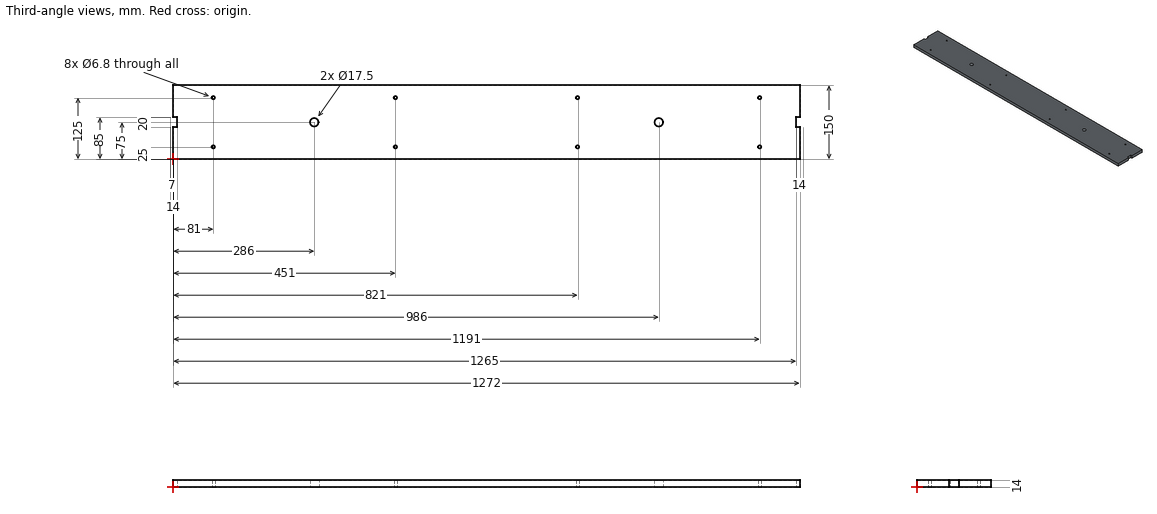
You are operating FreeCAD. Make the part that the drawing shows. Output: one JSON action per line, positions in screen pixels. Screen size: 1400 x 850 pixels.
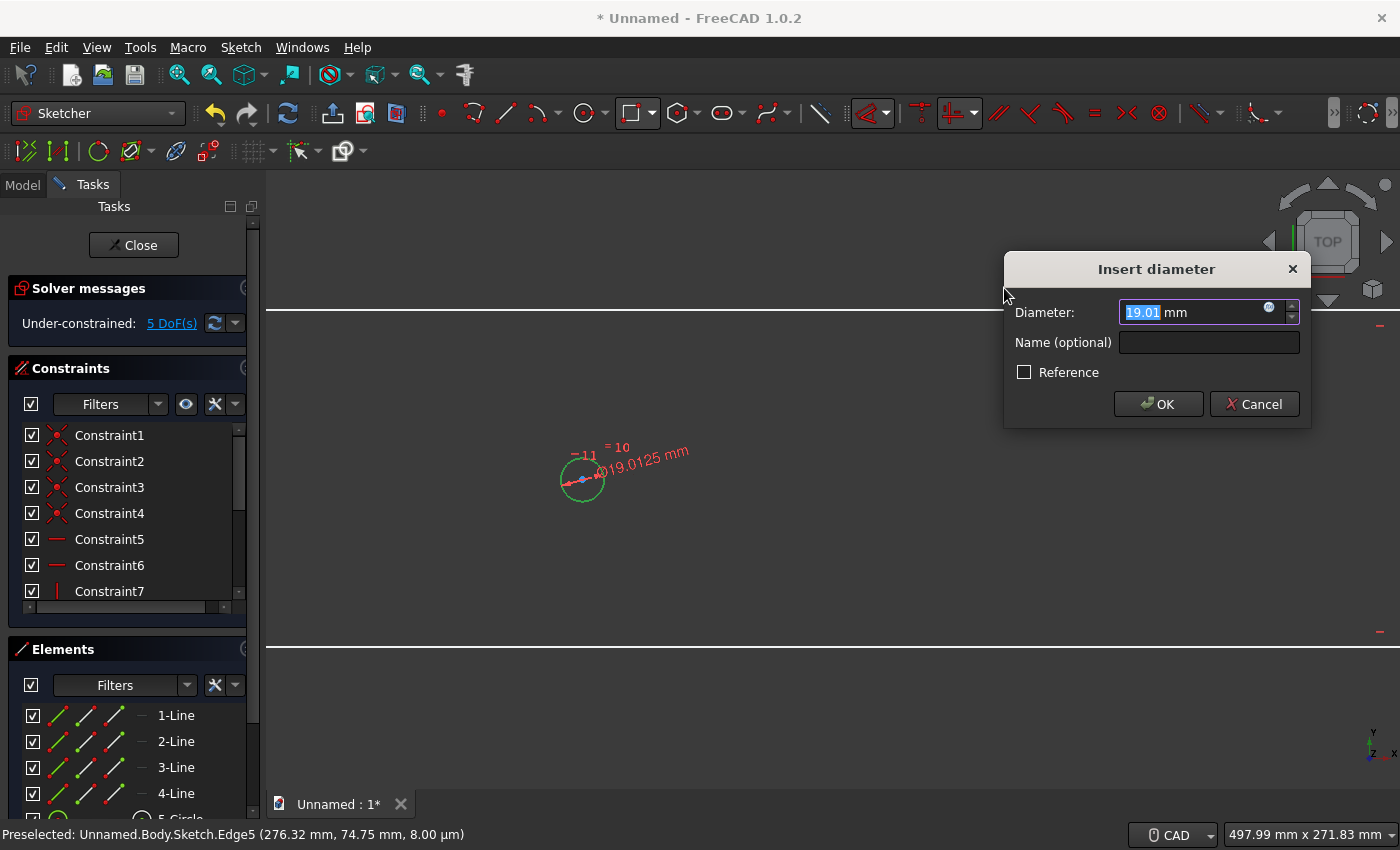
{"action": "type", "text": "17.5"}
{"action": "key", "text": "Return"}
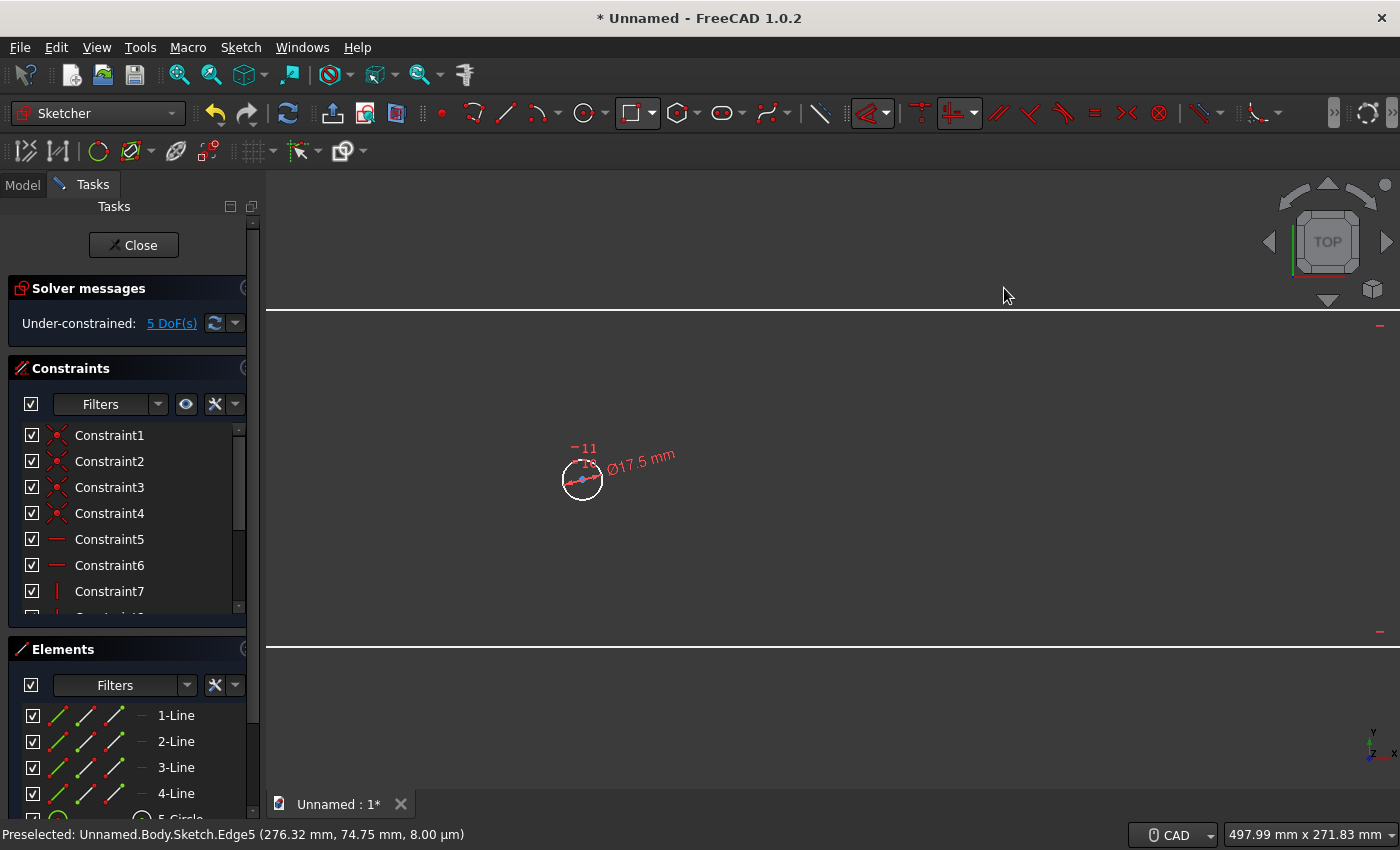
{"action": "scroll", "coordinate": [563, 480], "scroll_direction": "down", "scroll_amount": 7}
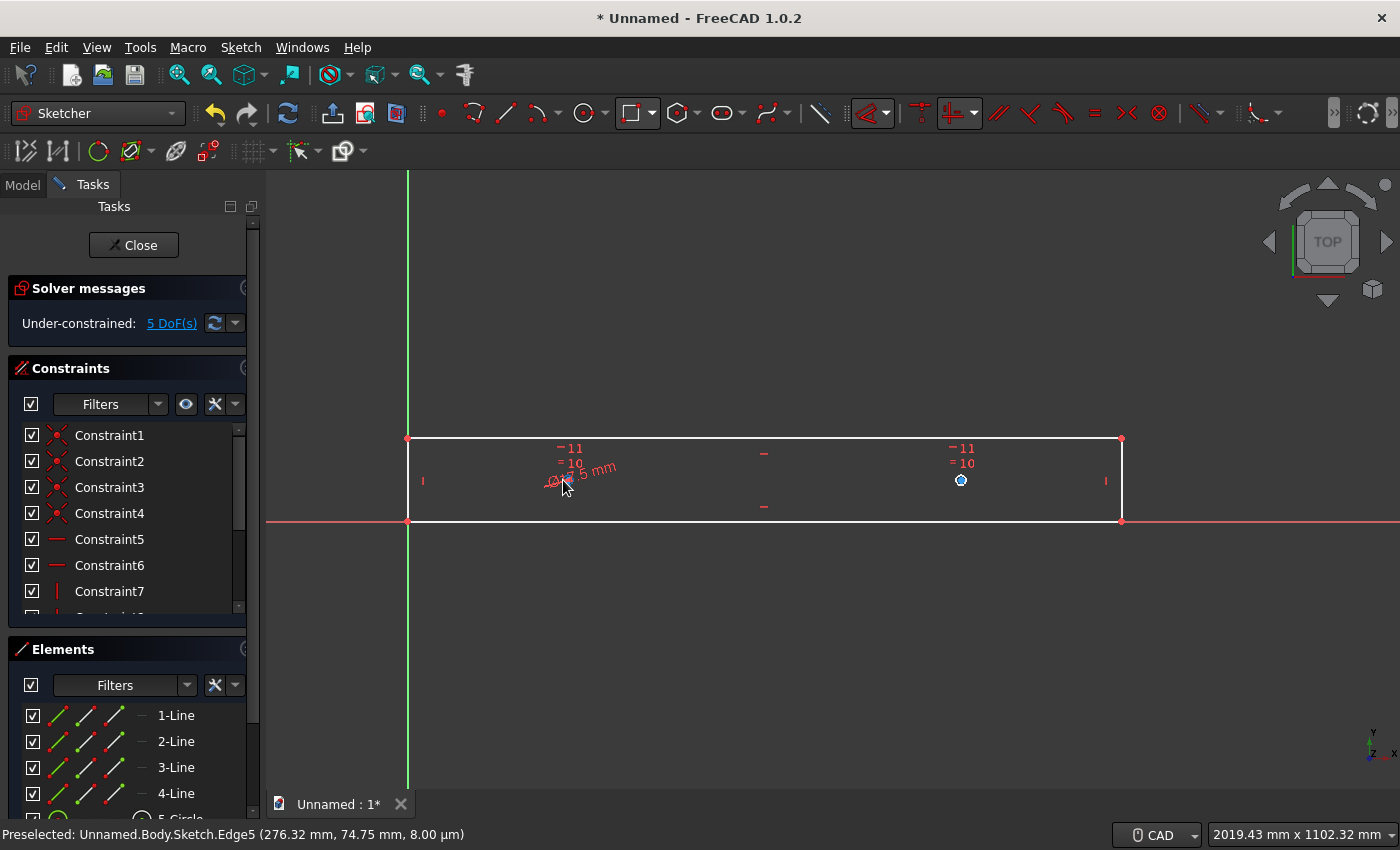
{"action": "left_click", "coordinate": [568, 480]}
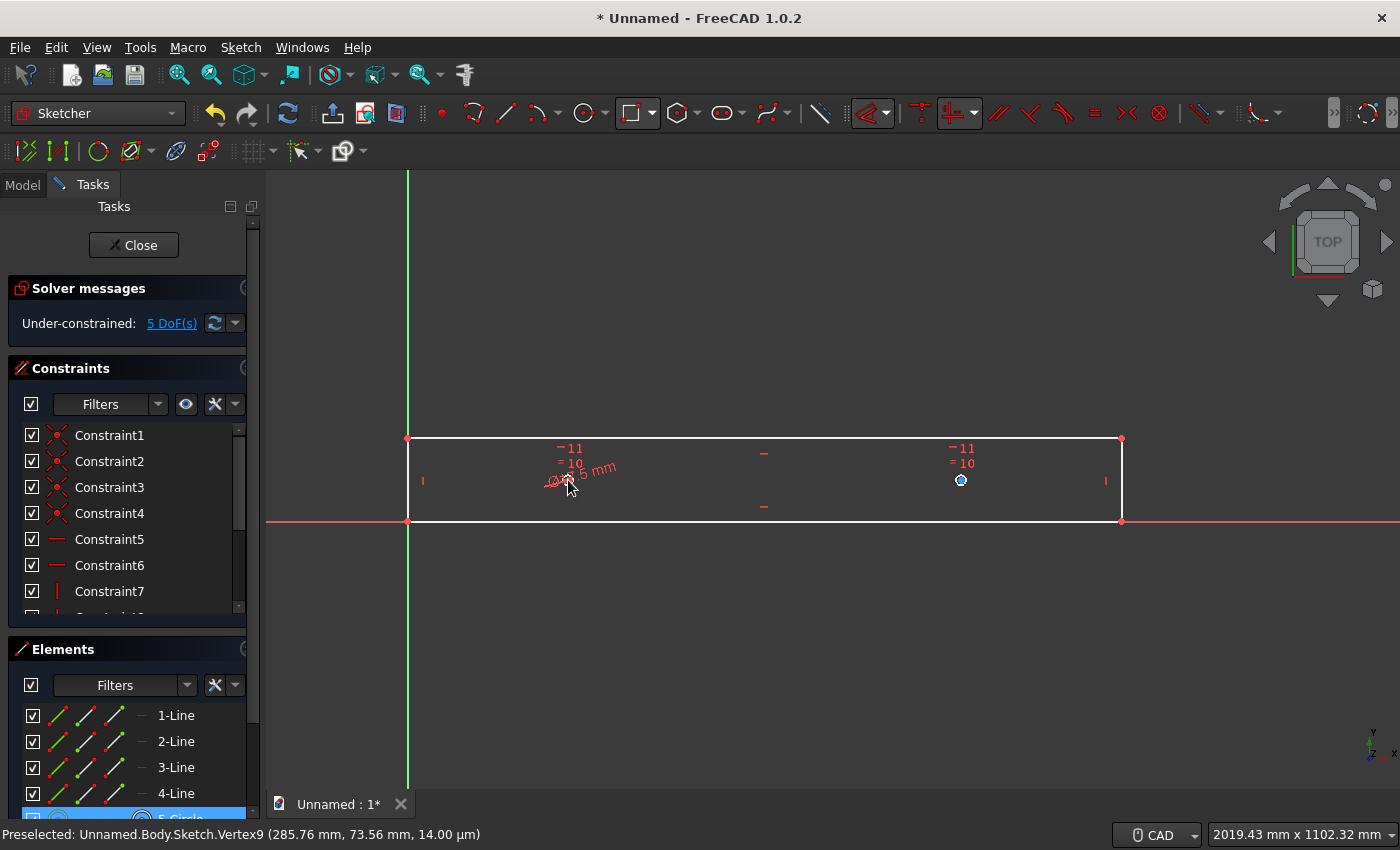
{"action": "left_click", "coordinate": [888, 114]}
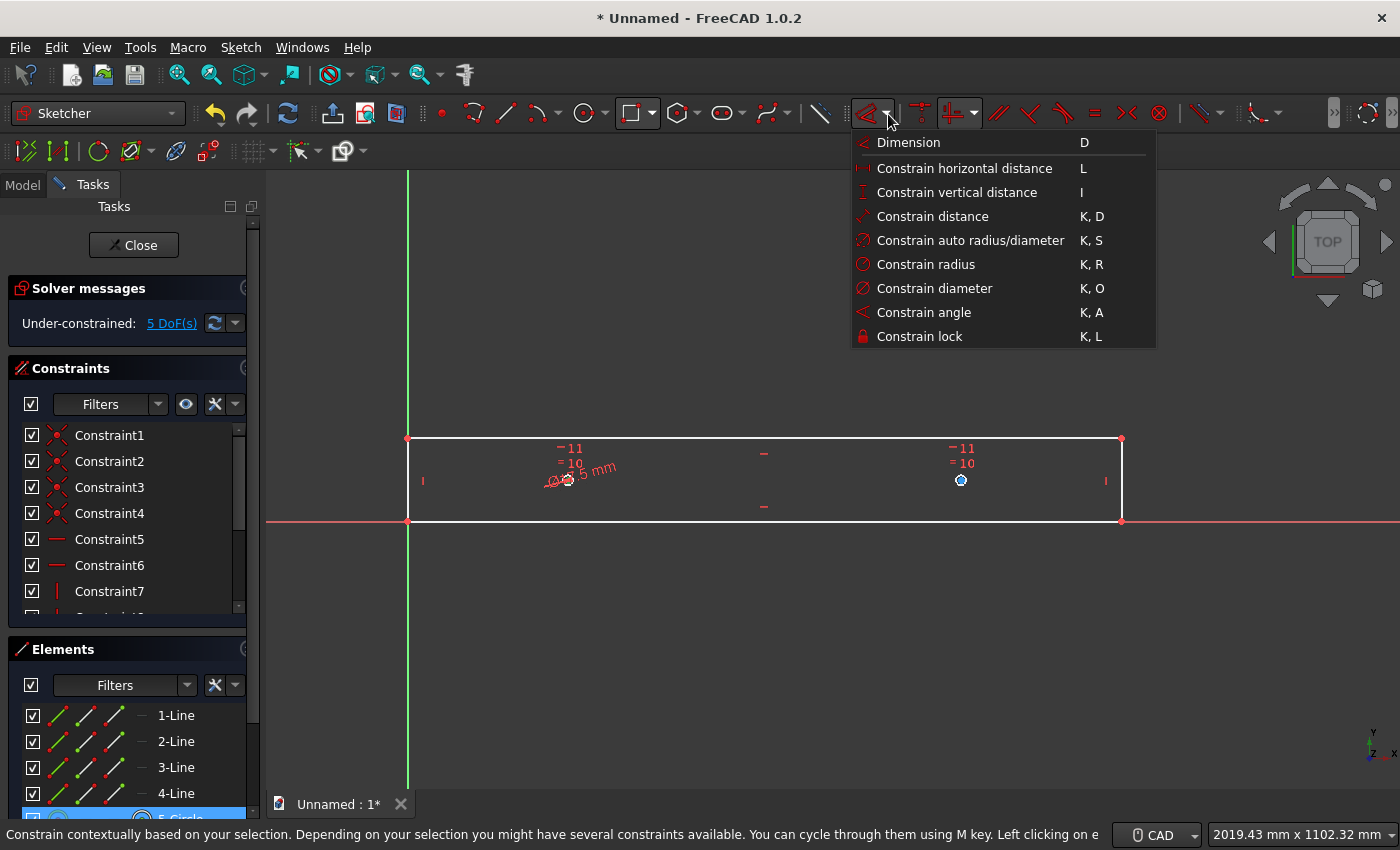
{"action": "left_click", "coordinate": [1004, 192]}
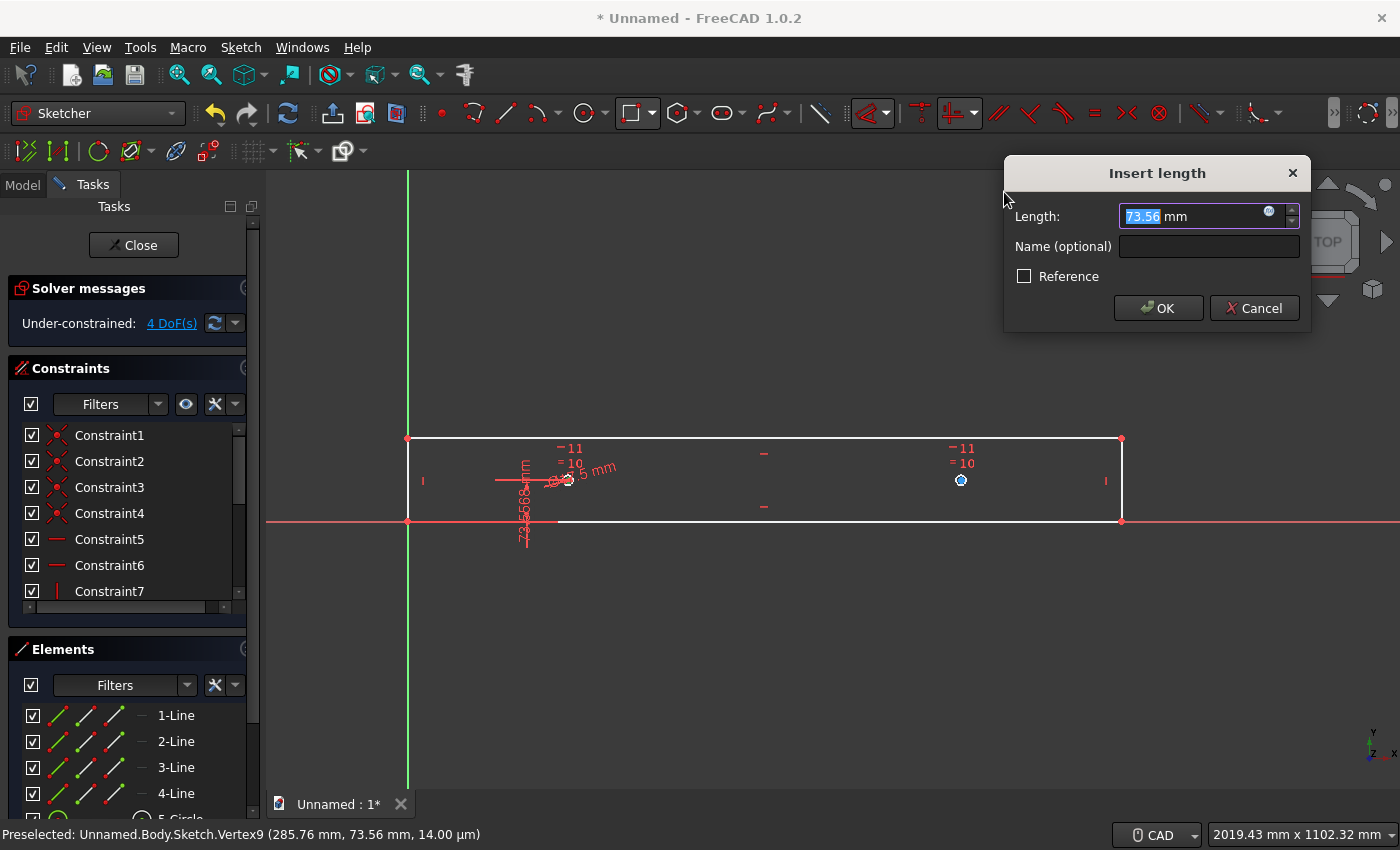
{"action": "type", "text": "75"}
{"action": "key", "text": "Return"}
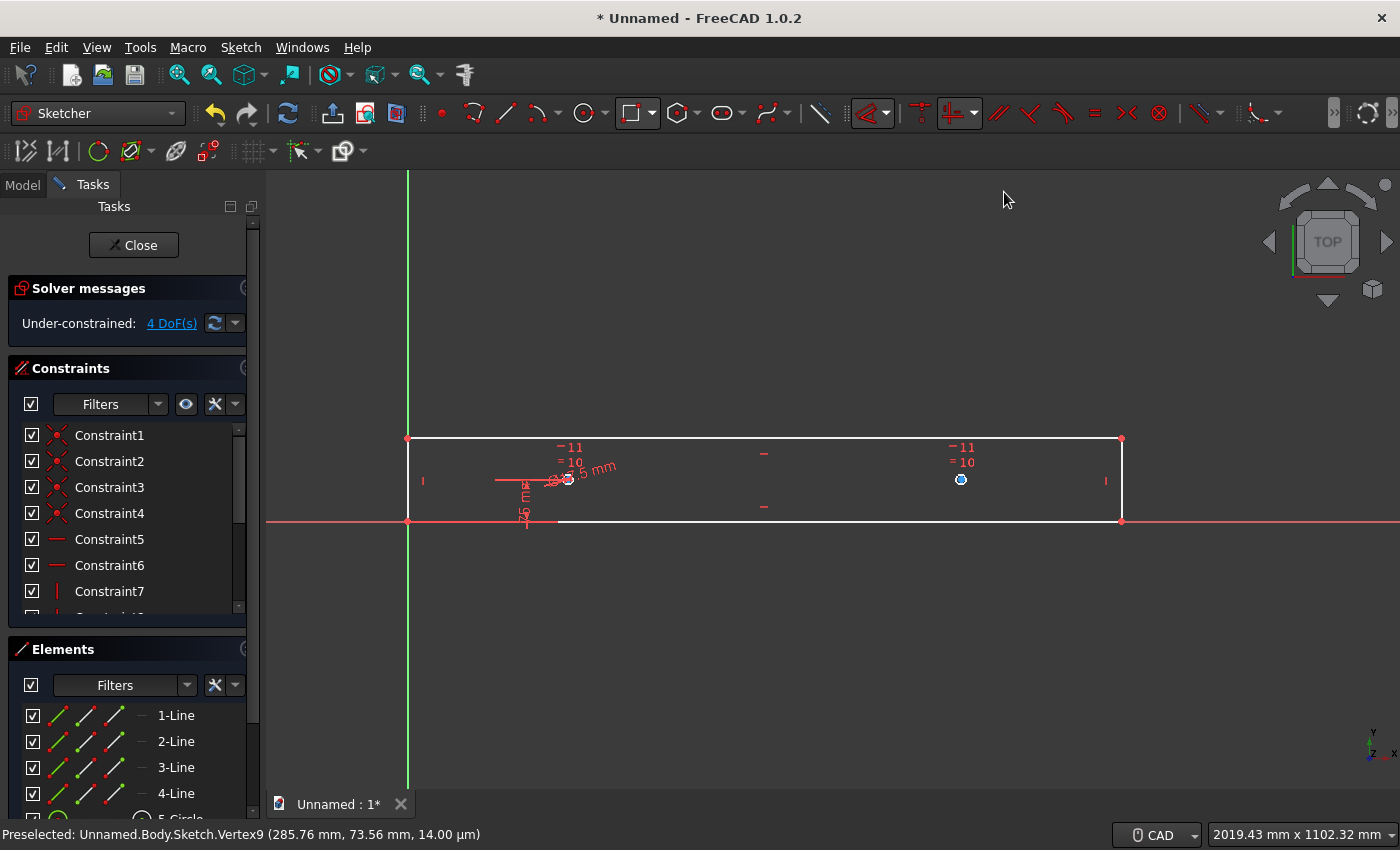
{"action": "left_click", "coordinate": [1122, 497]}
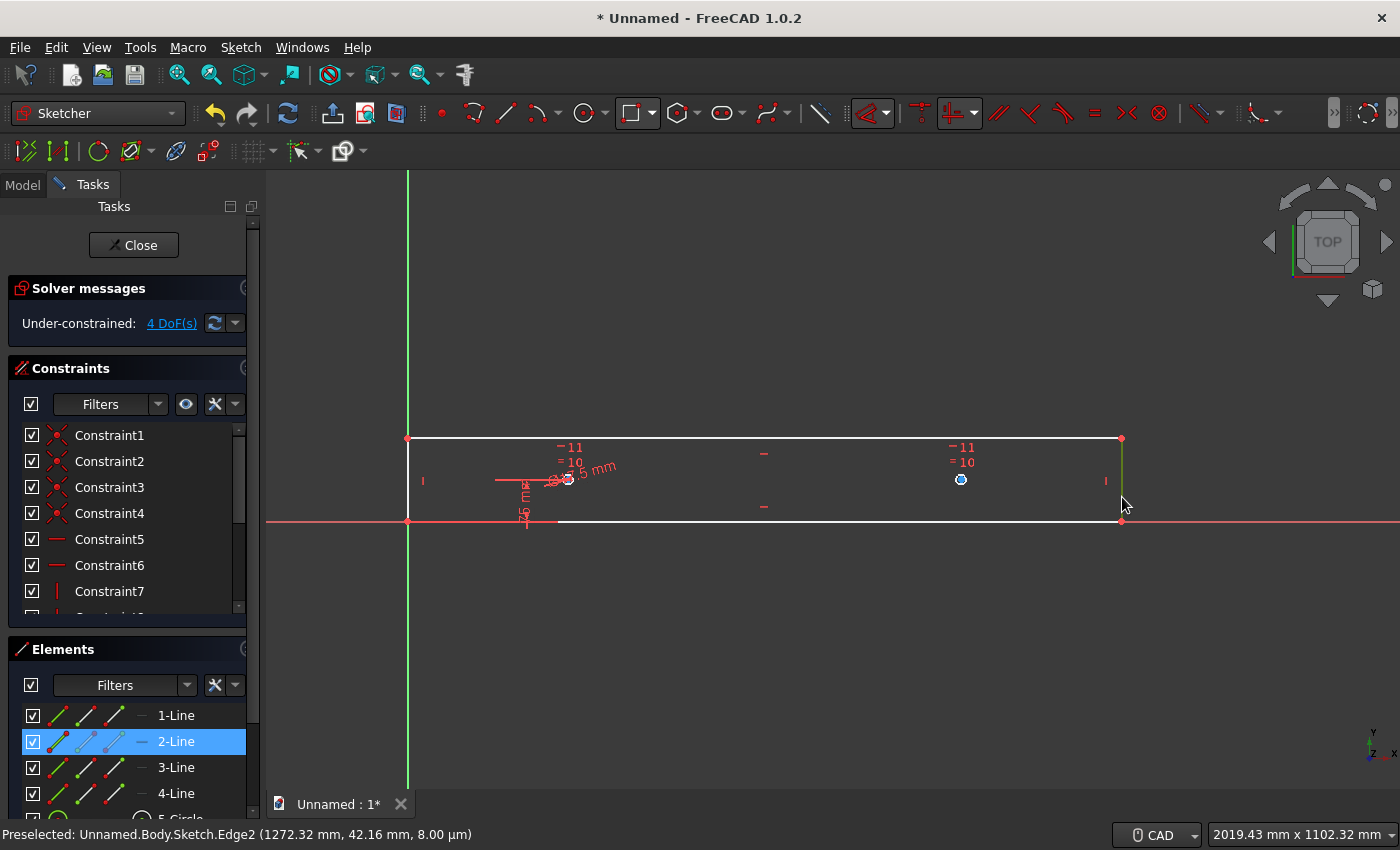
{"action": "left_click", "coordinate": [888, 114]}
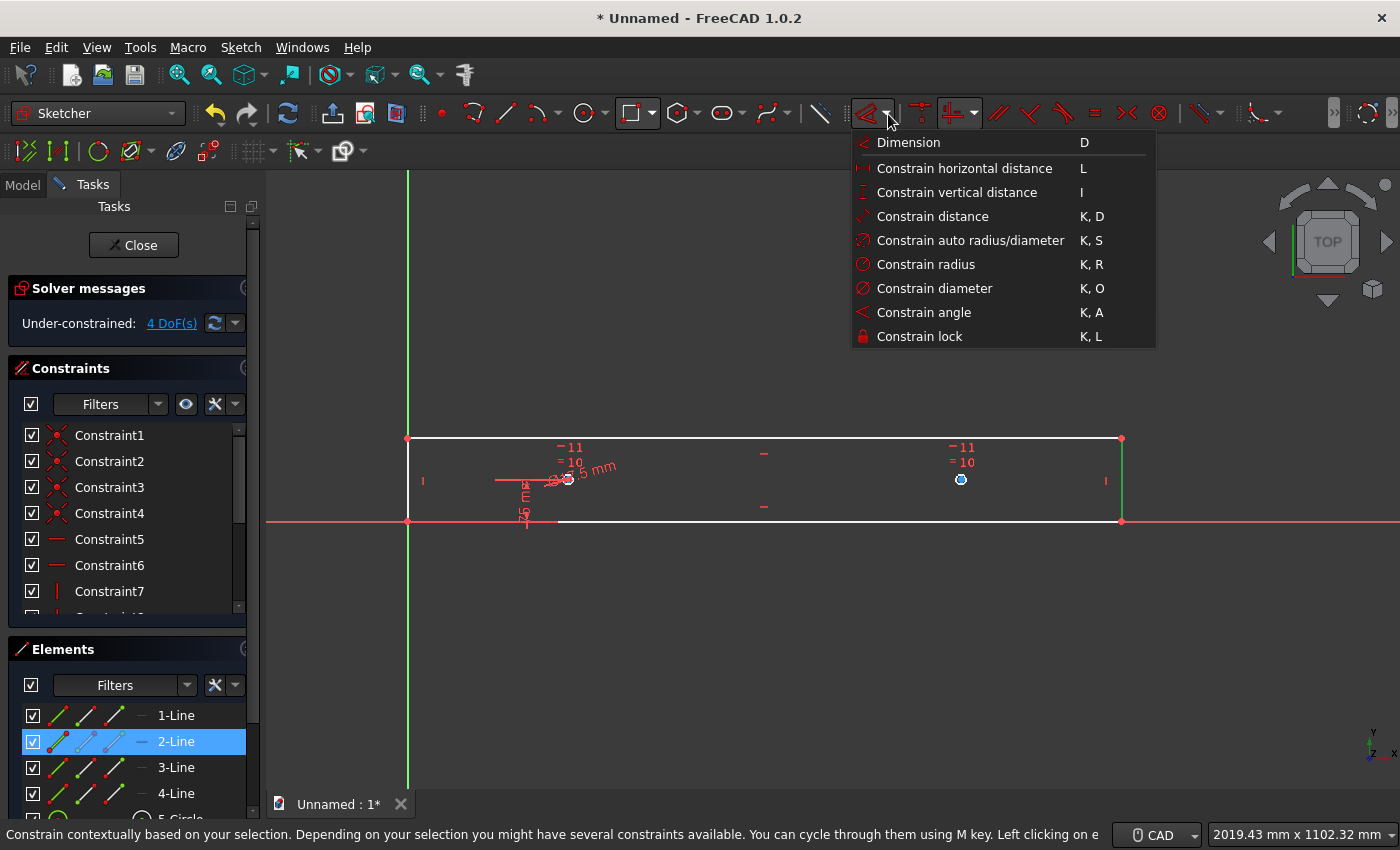
{"action": "left_click", "coordinate": [1004, 192]}